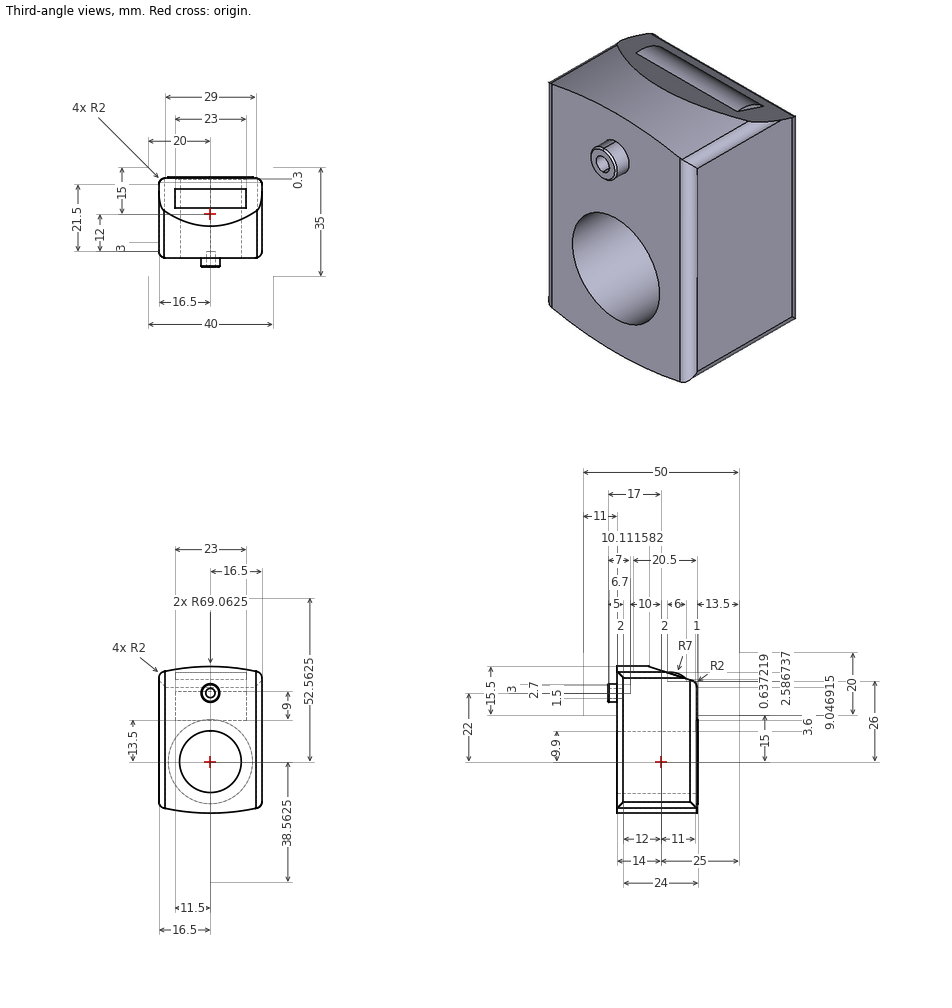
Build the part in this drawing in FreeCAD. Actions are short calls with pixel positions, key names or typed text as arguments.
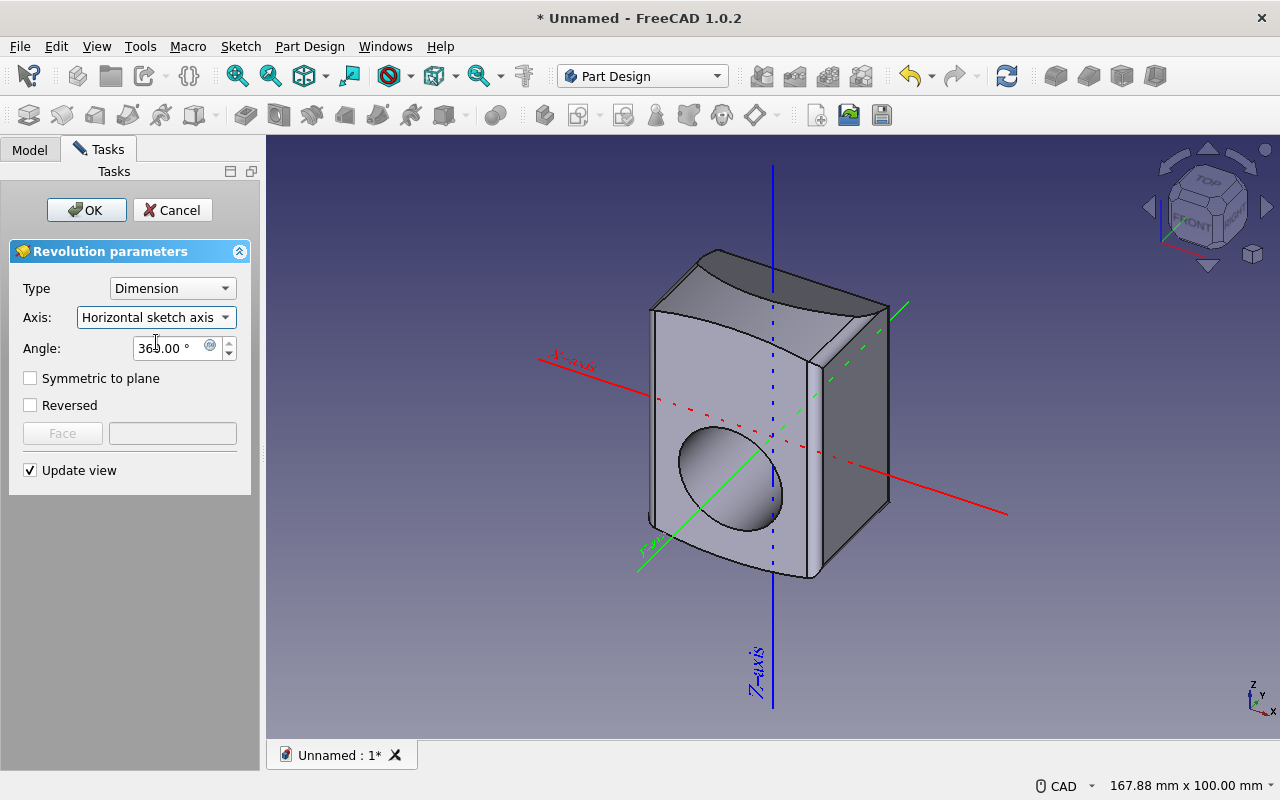
click(87, 210)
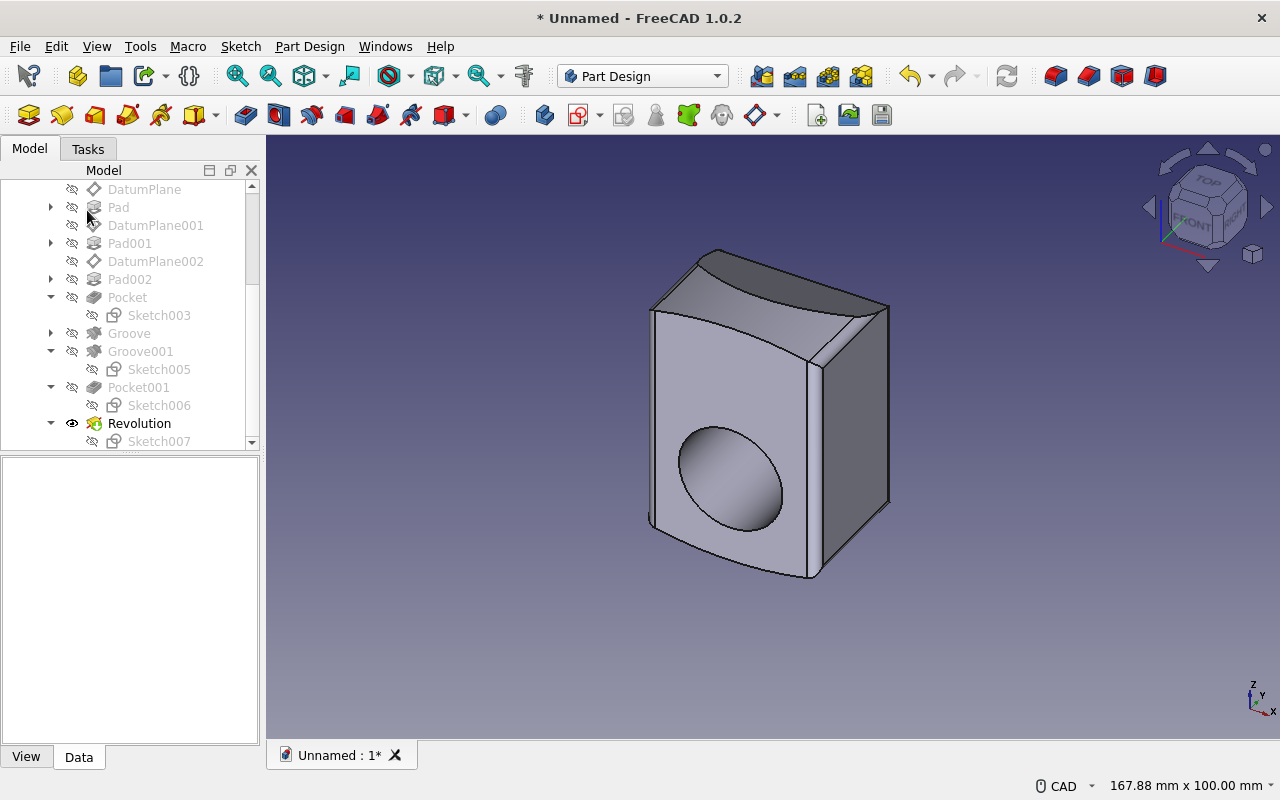
click(578, 116)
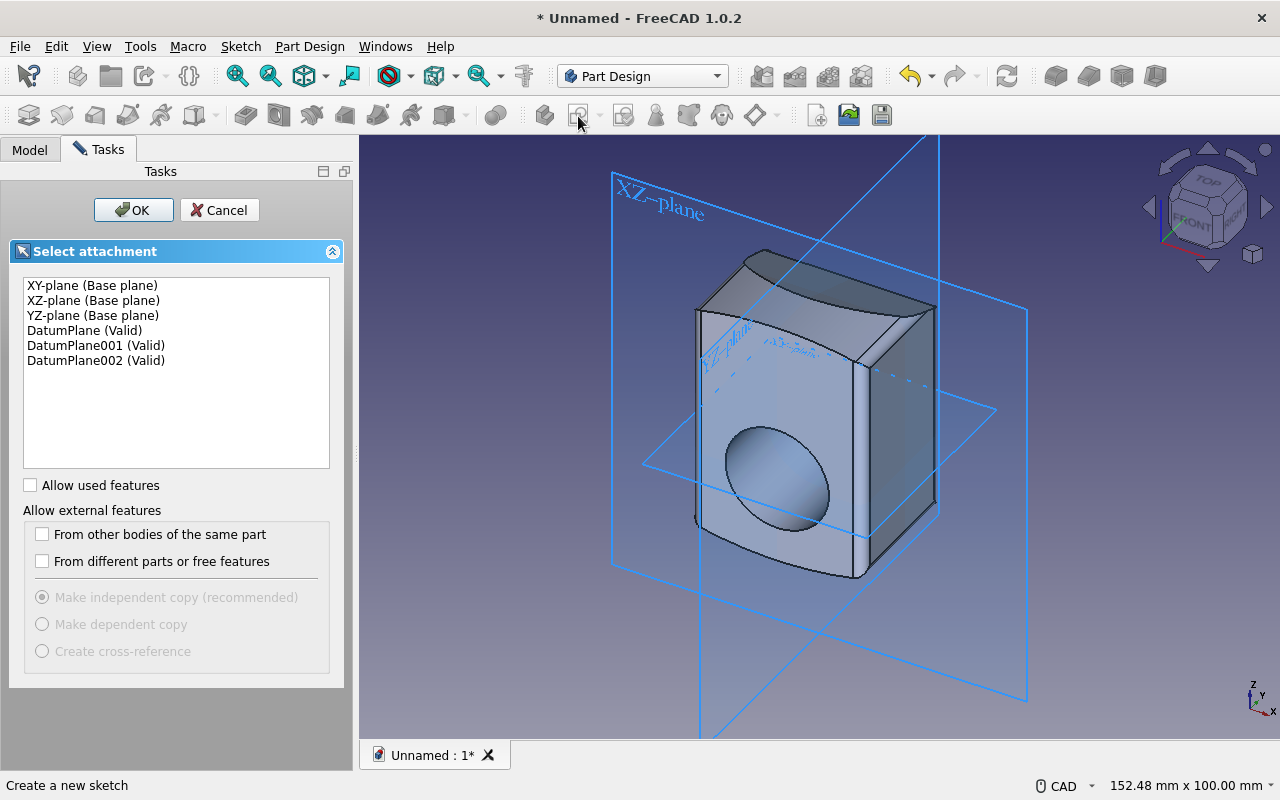
click(84, 316)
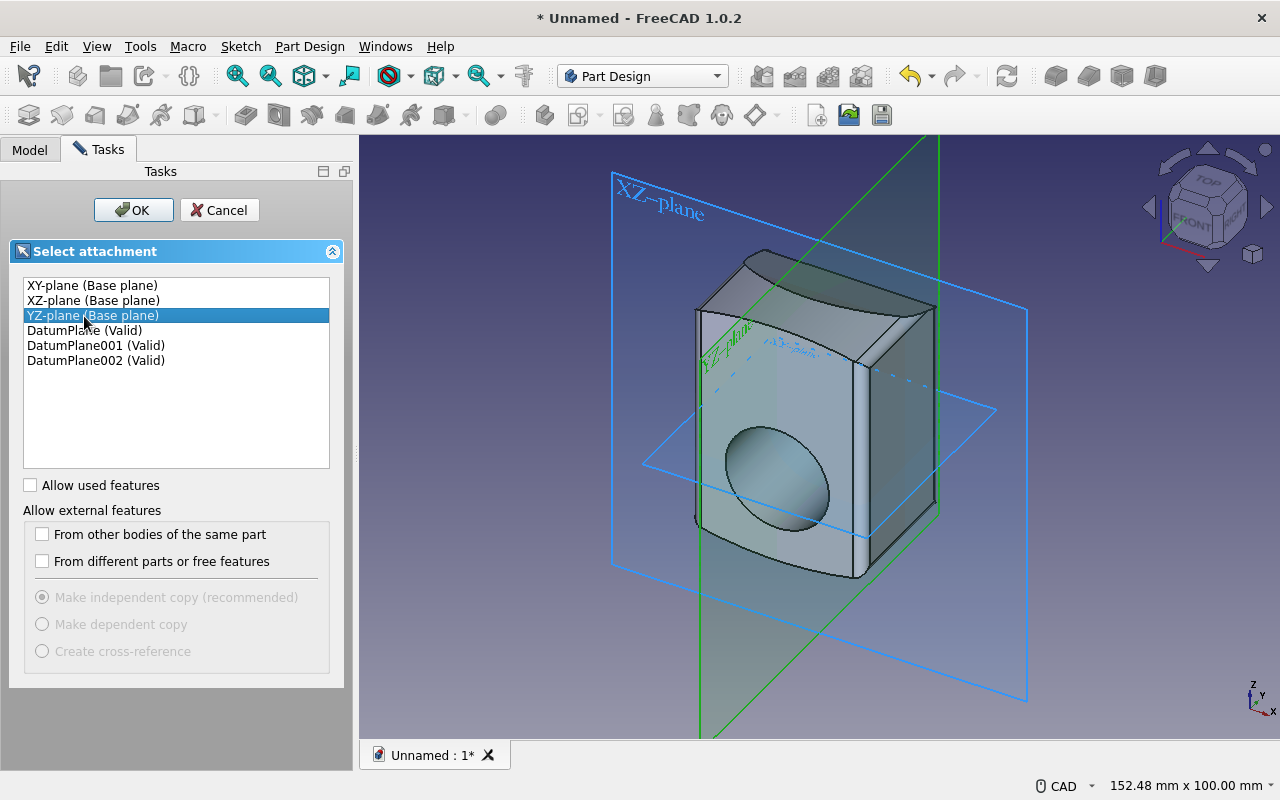
click(134, 210)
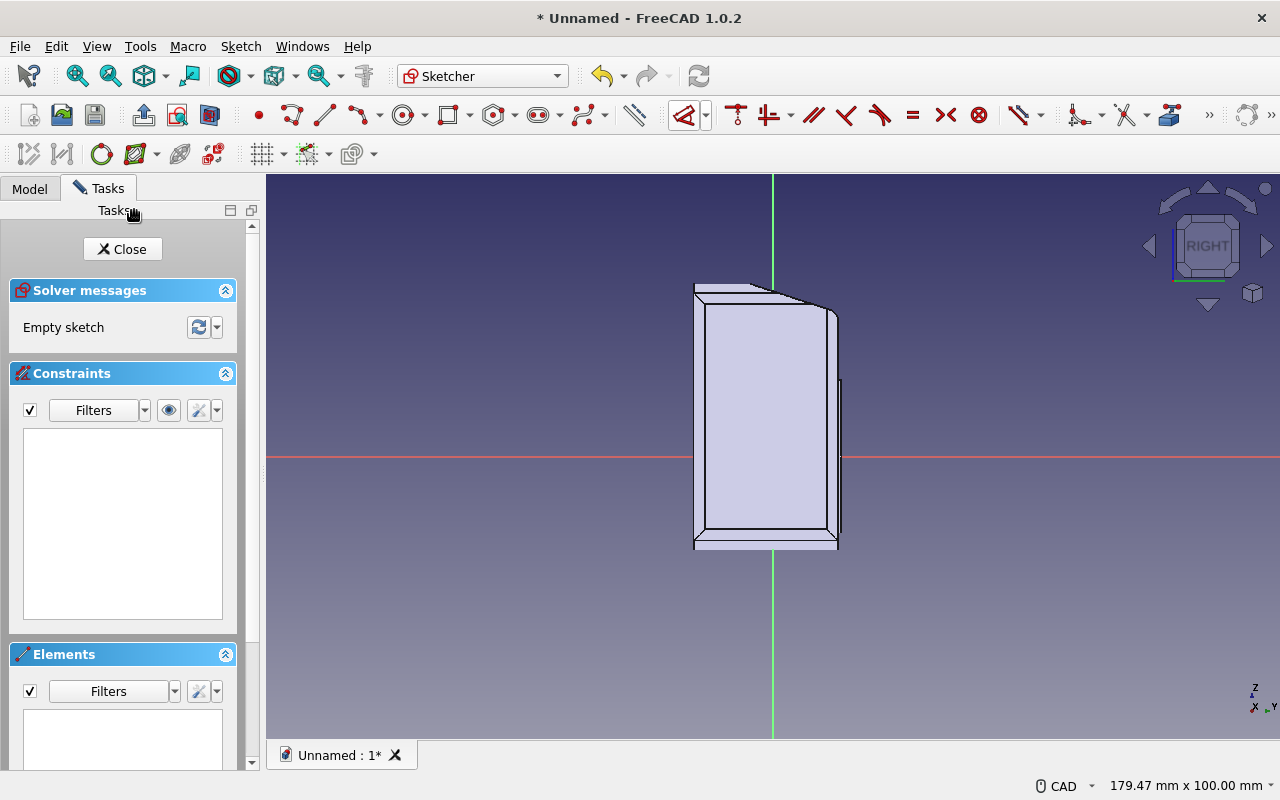
click(210, 116)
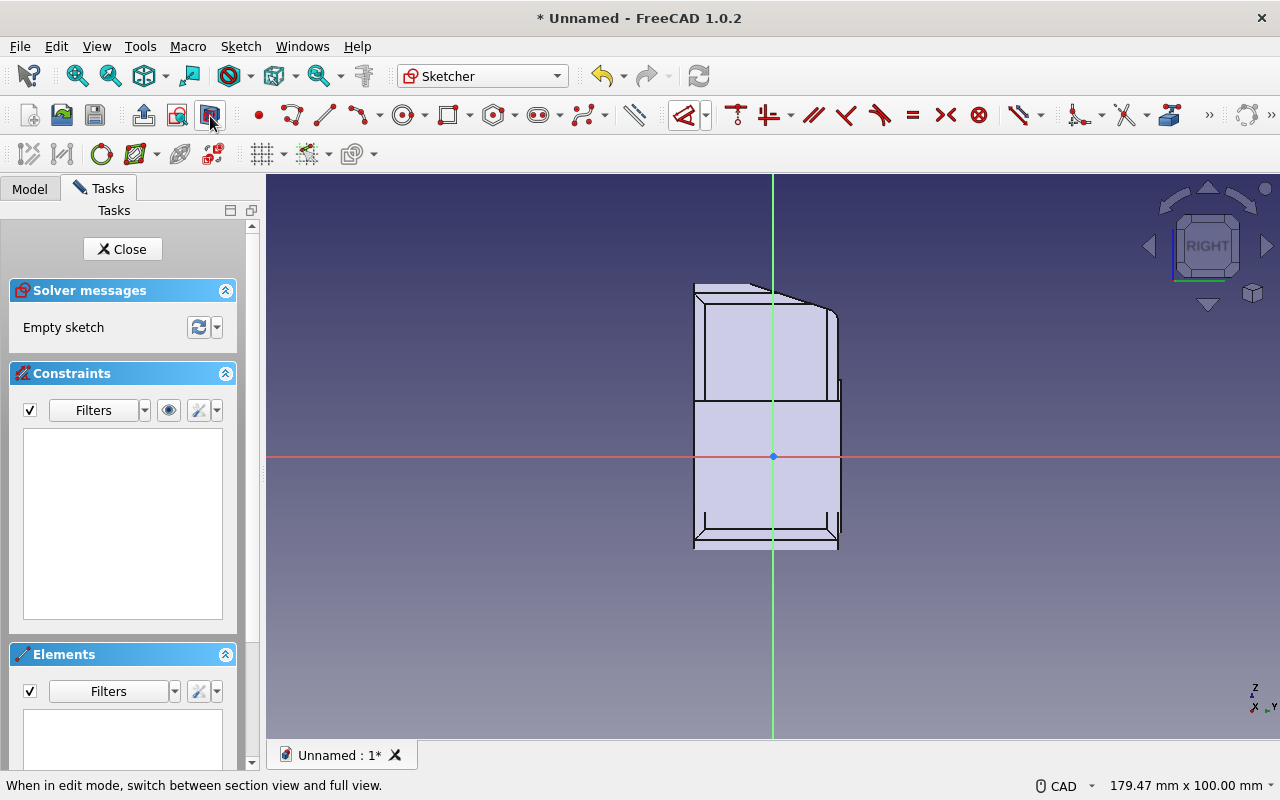
scroll(687, 310, up, 12)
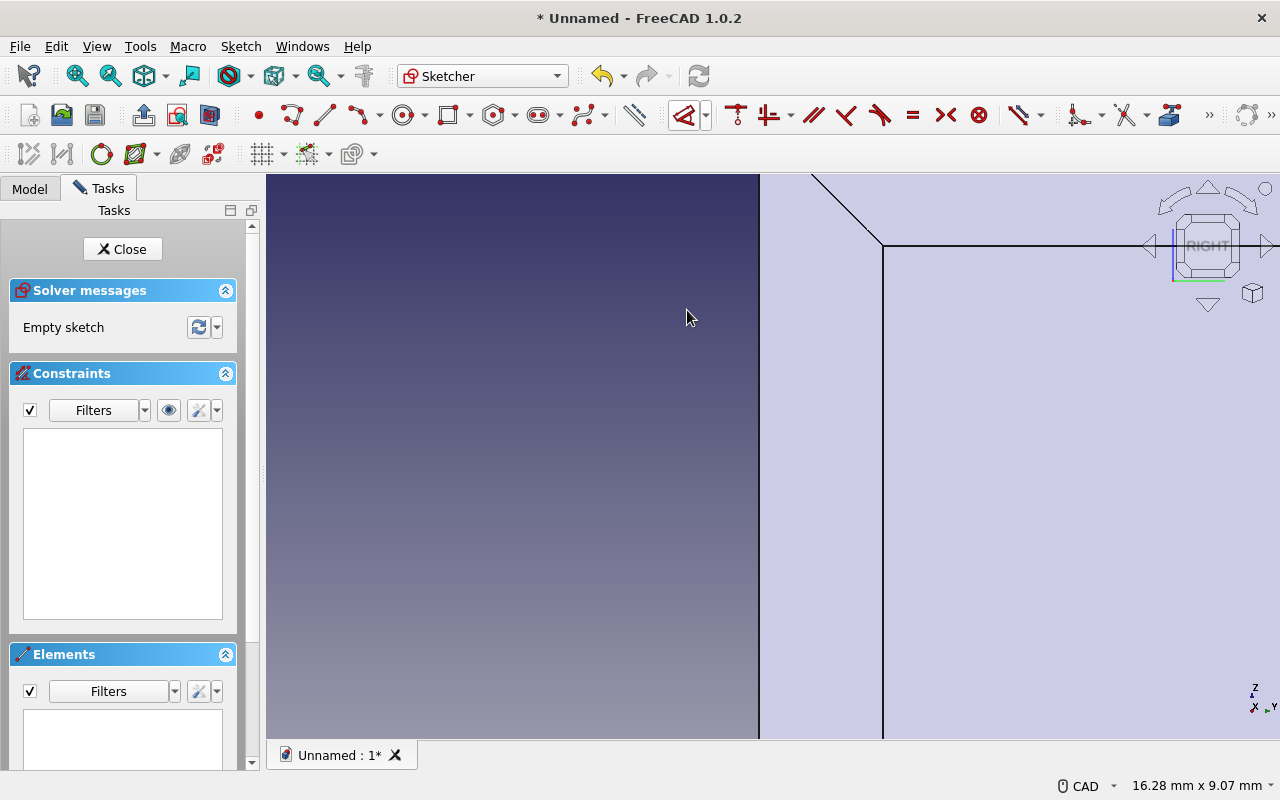
click(292, 116)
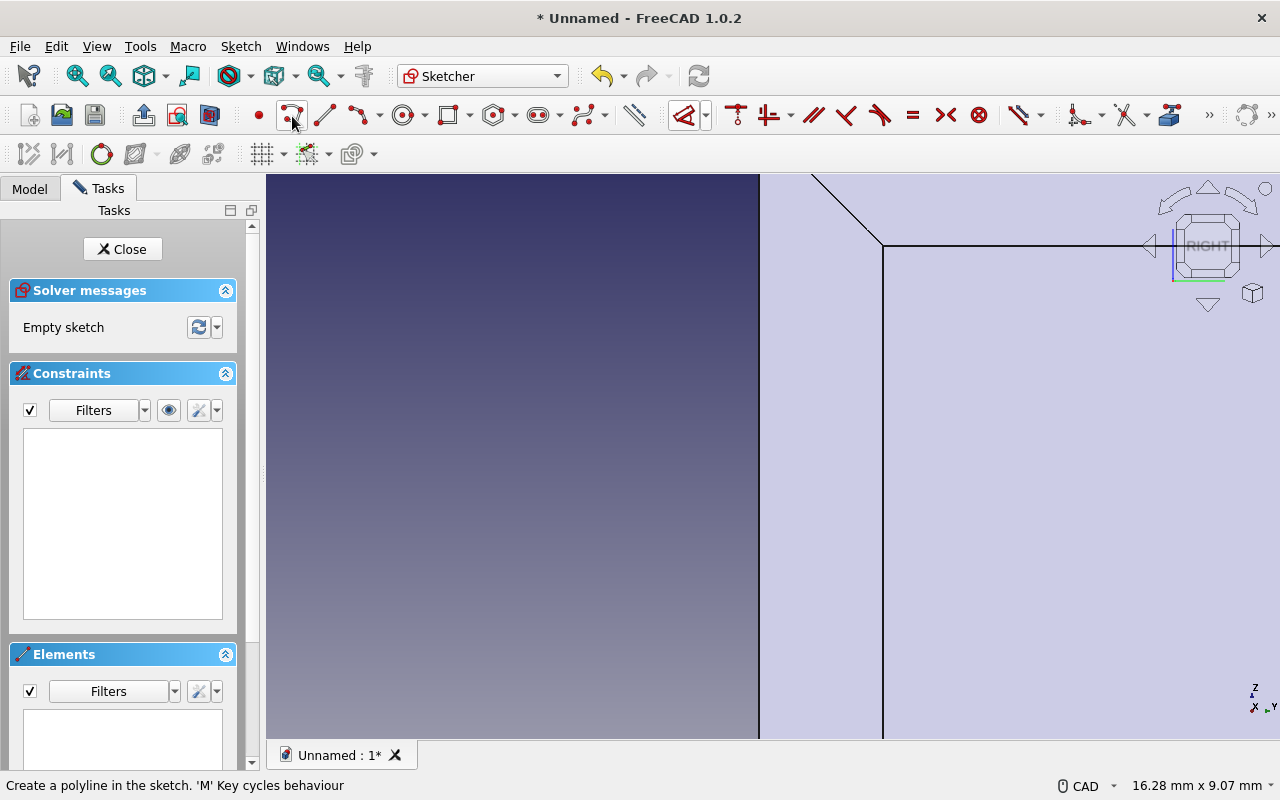
click(1008, 552)
click(1008, 365)
click(591, 365)
click(572, 384)
click(572, 552)
click(1008, 553)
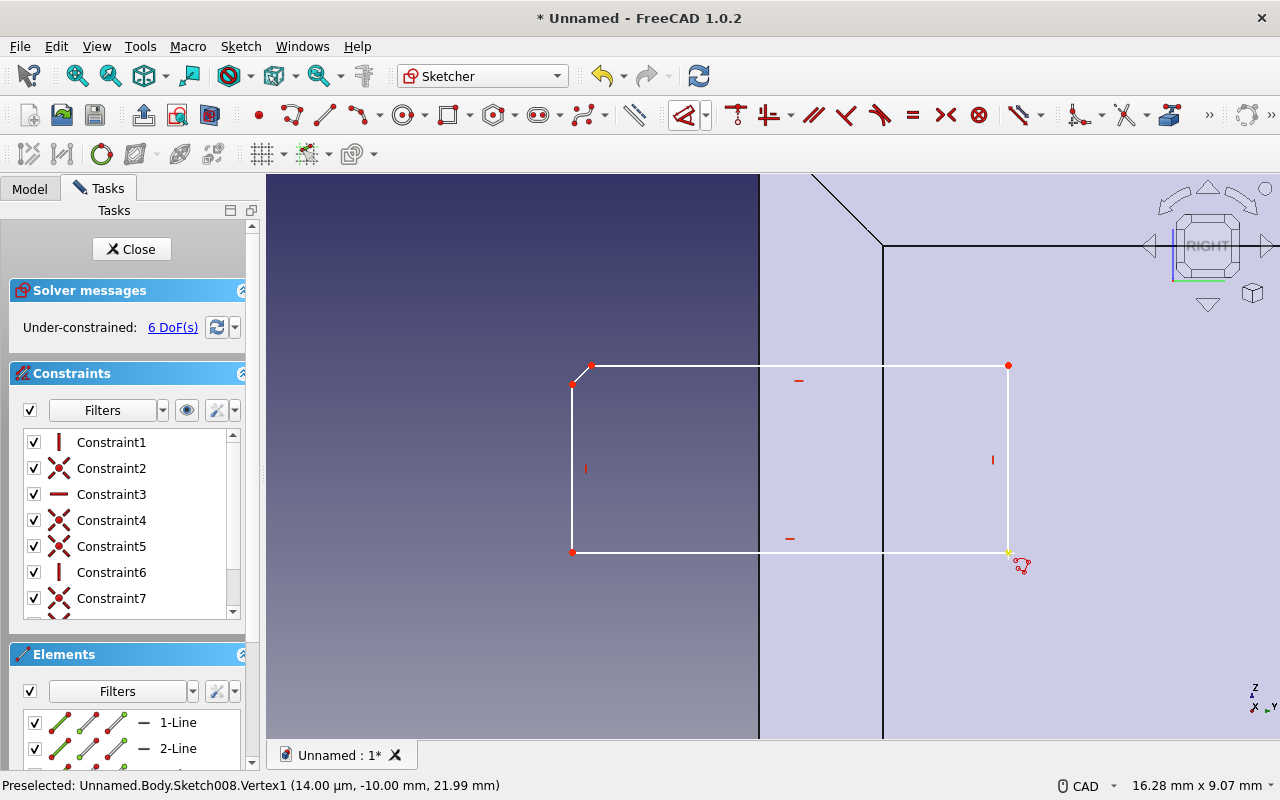
click(325, 116)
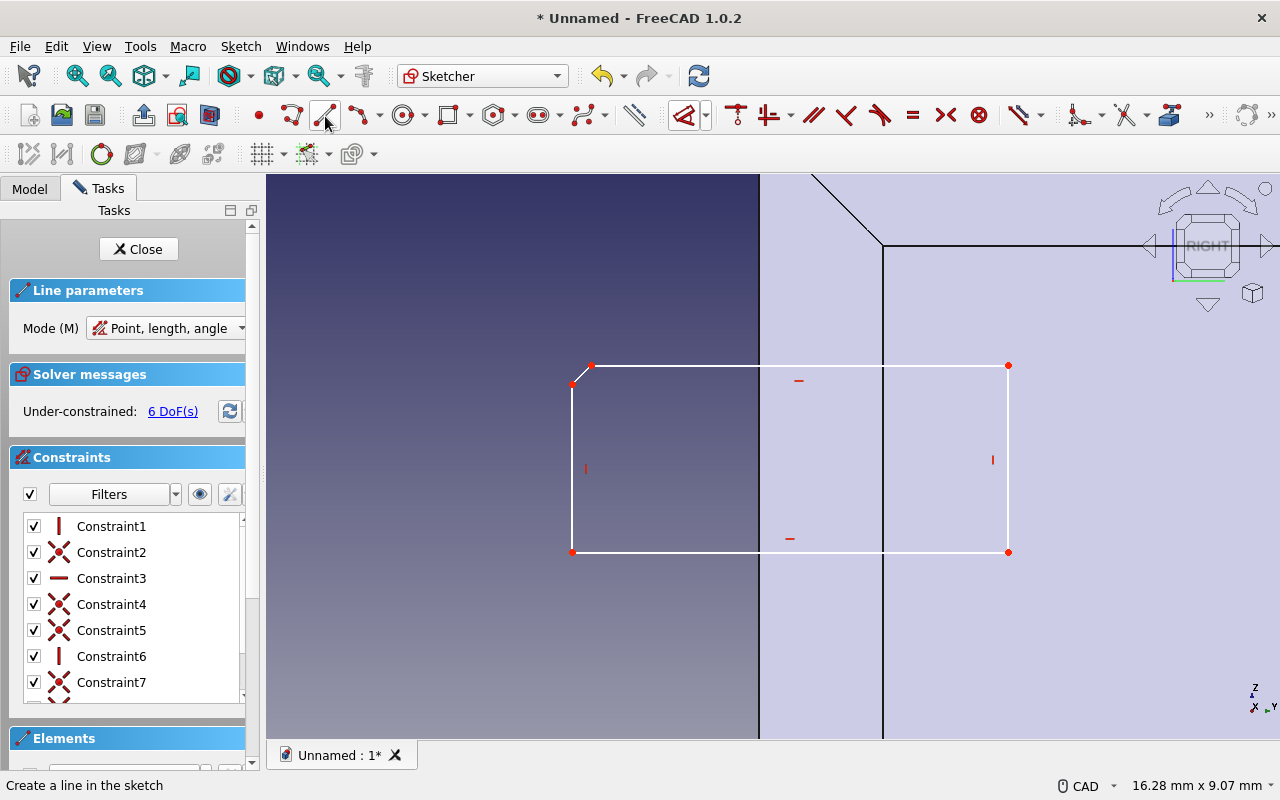
click(528, 552)
click(398, 552)
key(Escape)